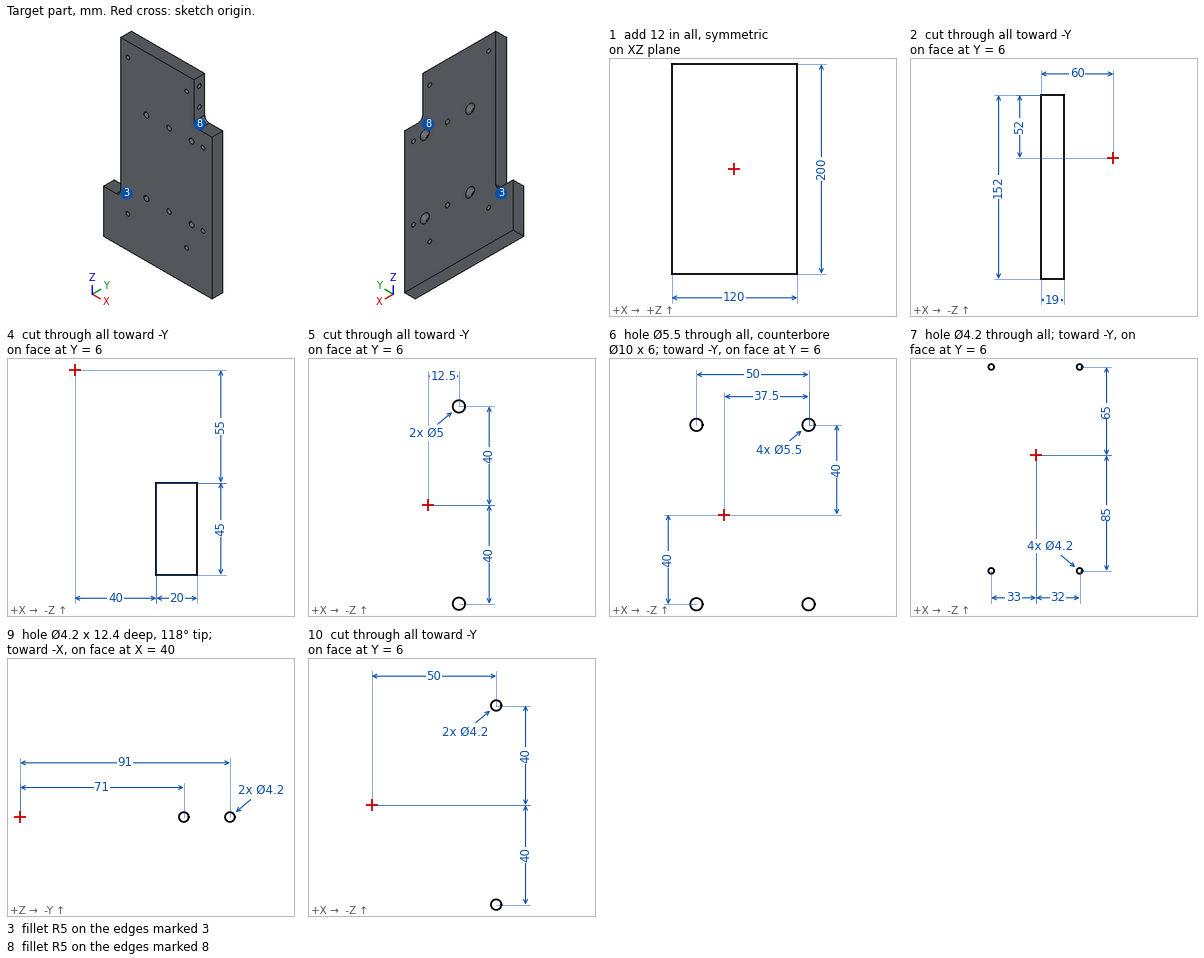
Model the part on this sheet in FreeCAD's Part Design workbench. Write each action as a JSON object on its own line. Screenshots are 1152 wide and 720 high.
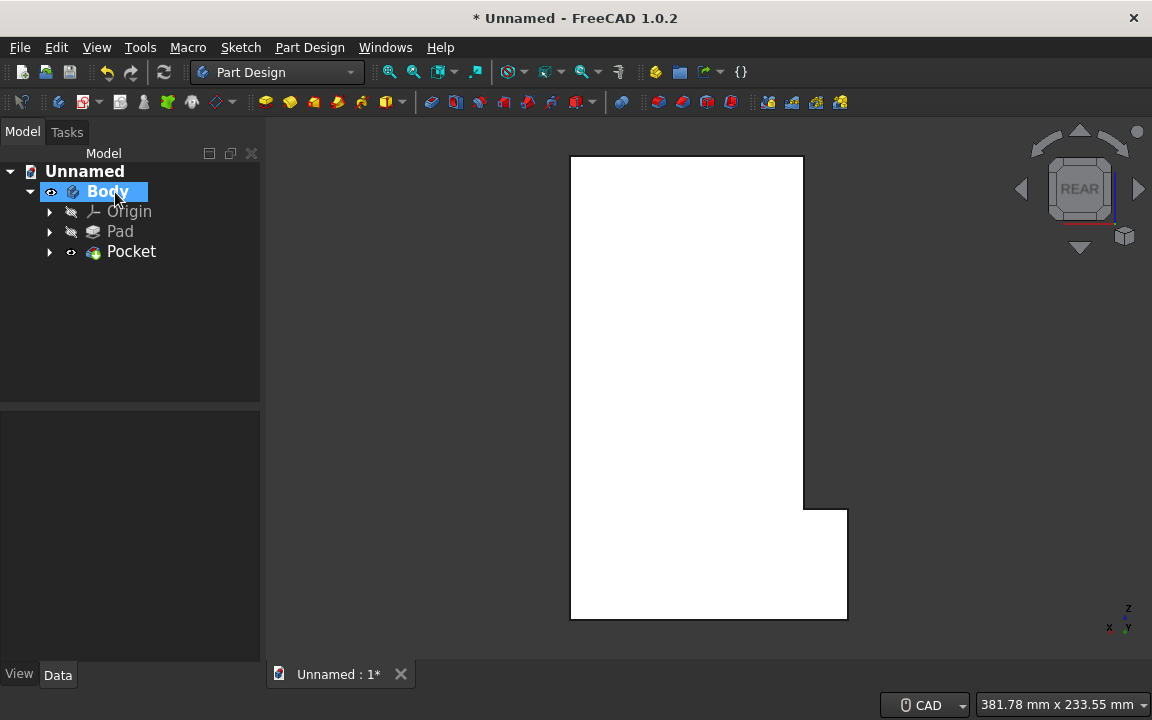
{"action": "key", "text": "0"}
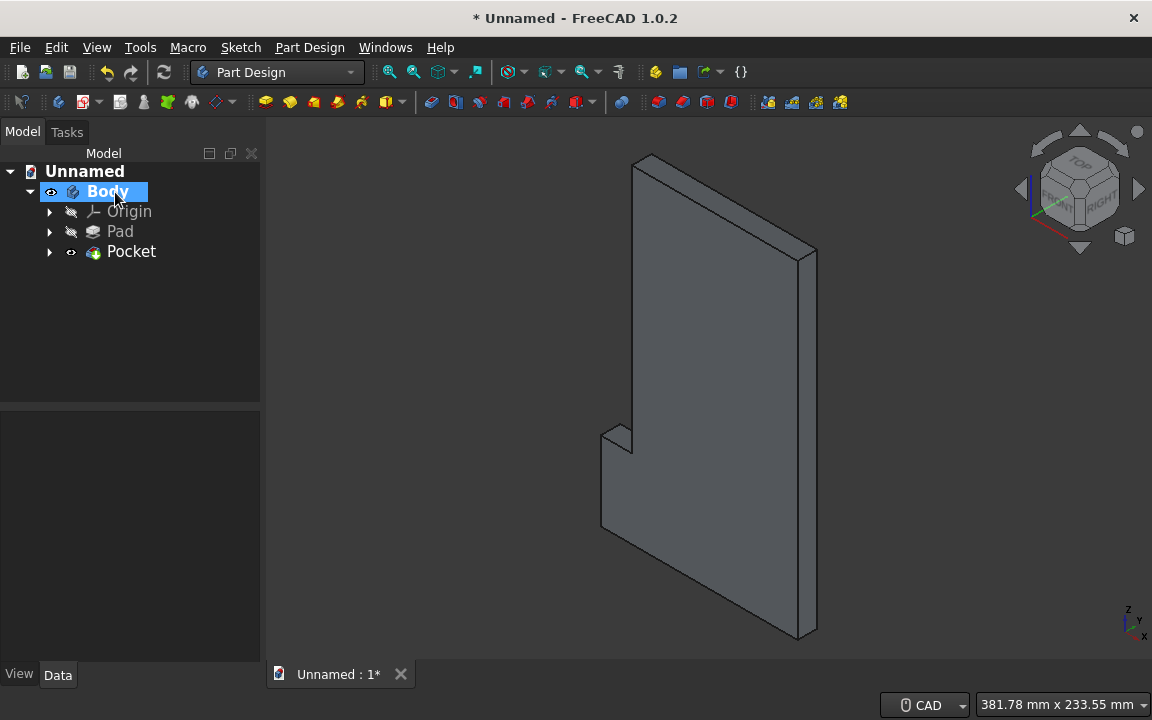
{"action": "key", "text": "2"}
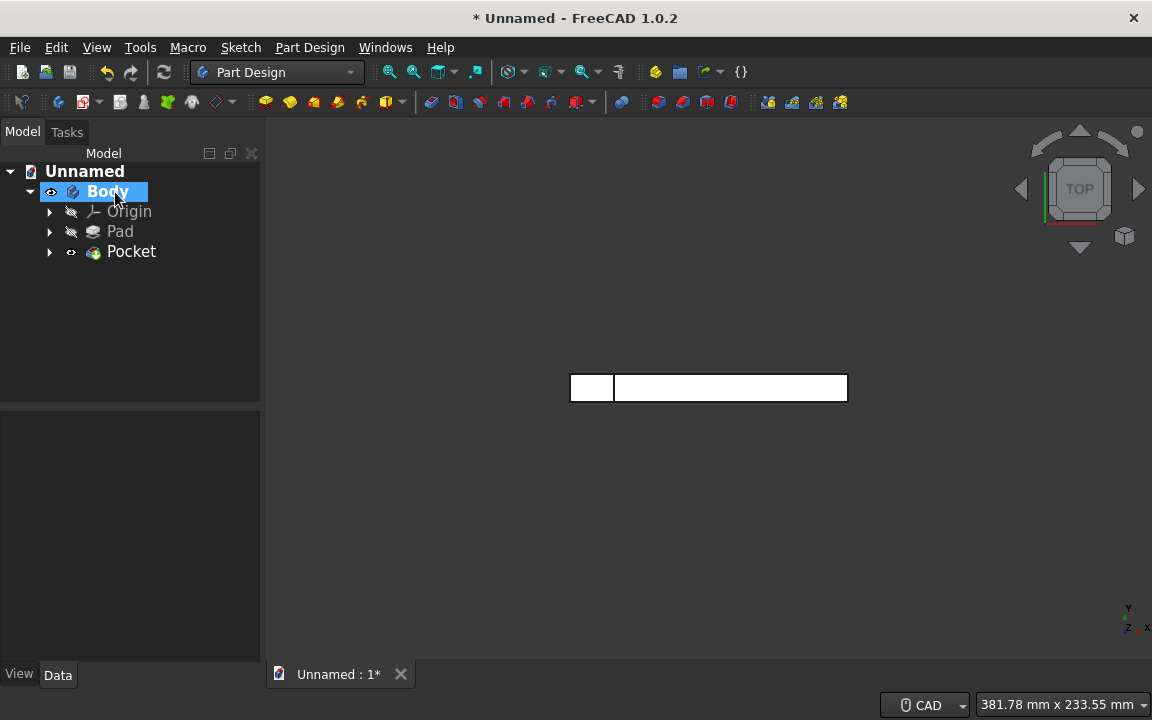
{"action": "left_click", "coordinate": [390, 72]}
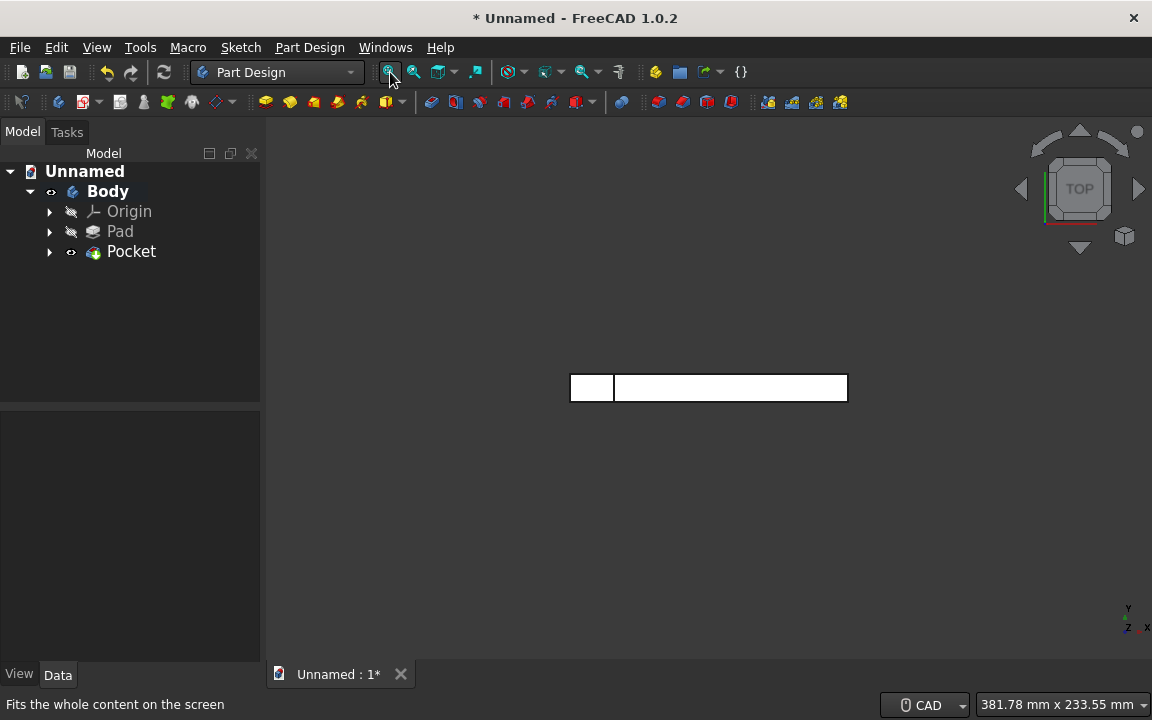
{"action": "key", "text": "1"}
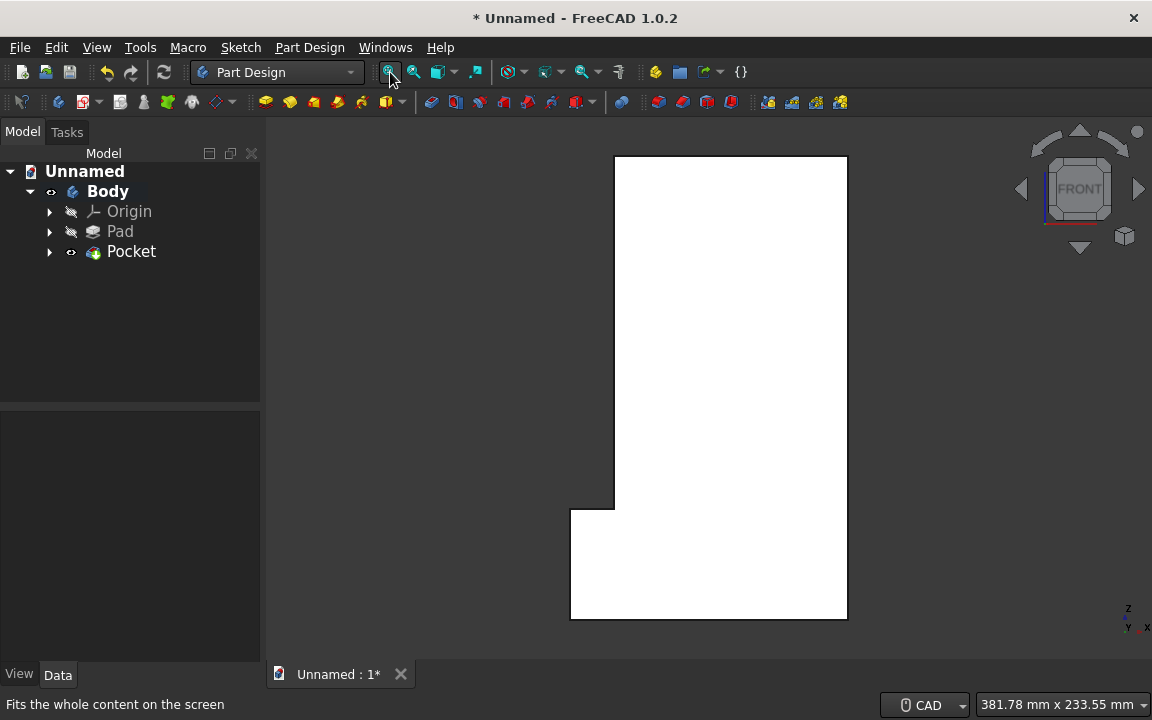
{"action": "key", "text": "3"}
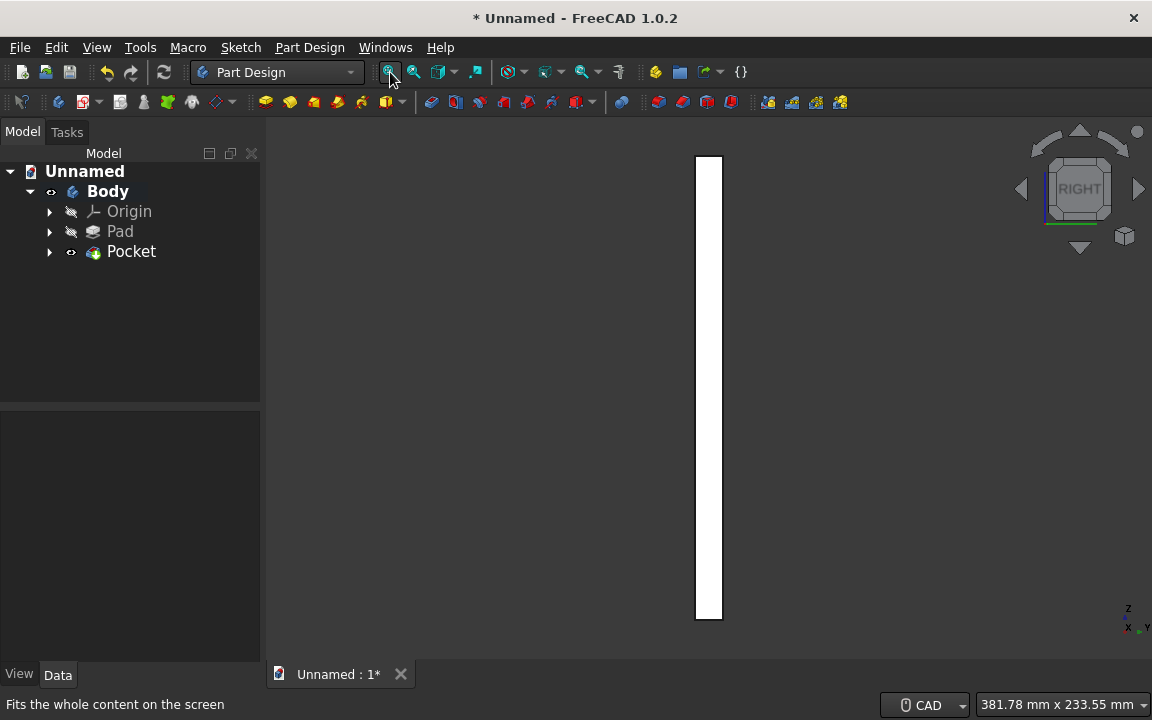
{"action": "key", "text": "5"}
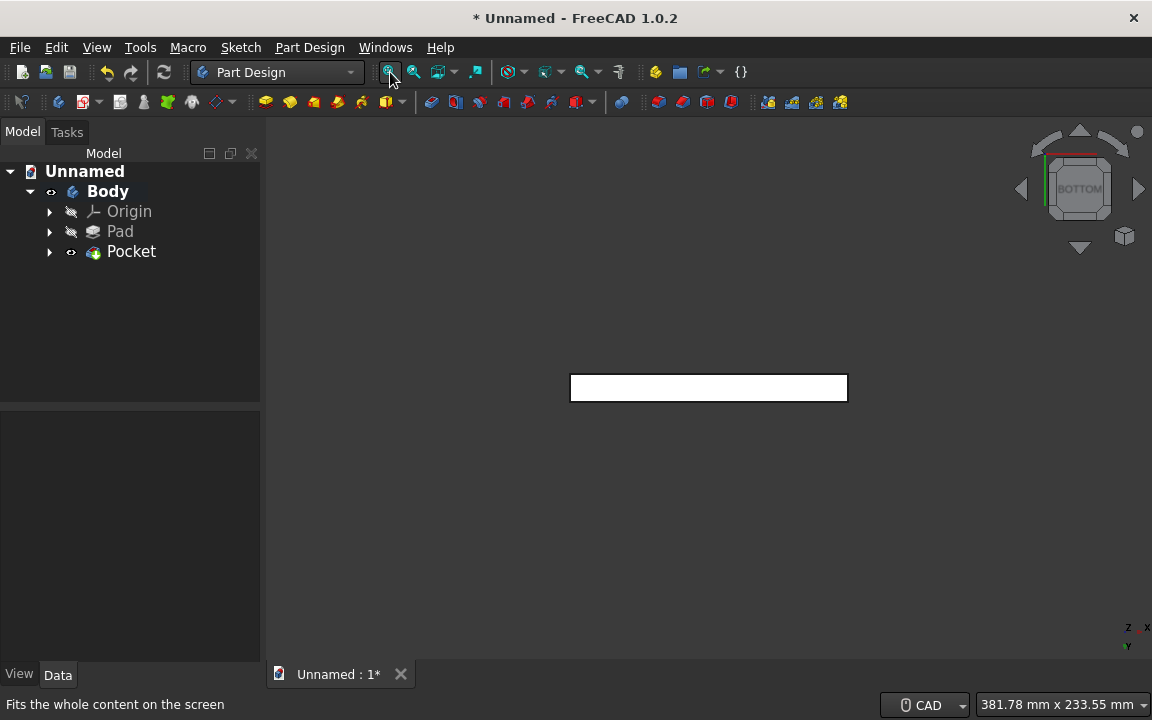
{"action": "left_click", "coordinate": [390, 72]}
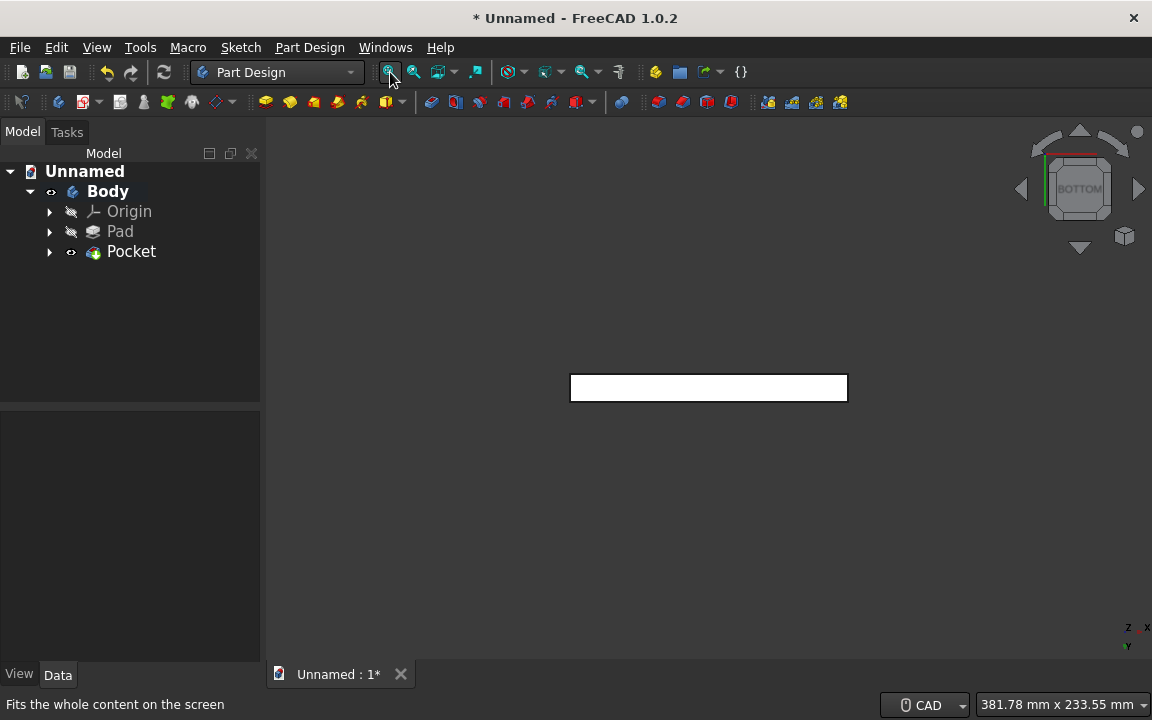
{"action": "key", "text": "4"}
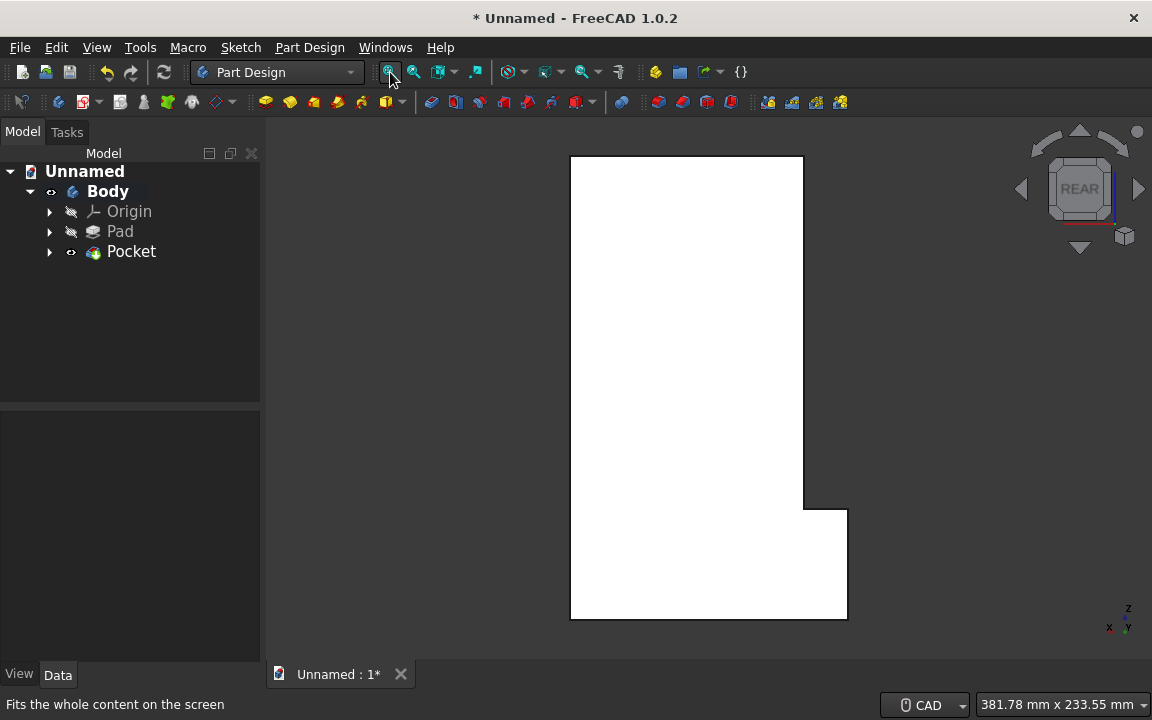
{"action": "key", "text": "6"}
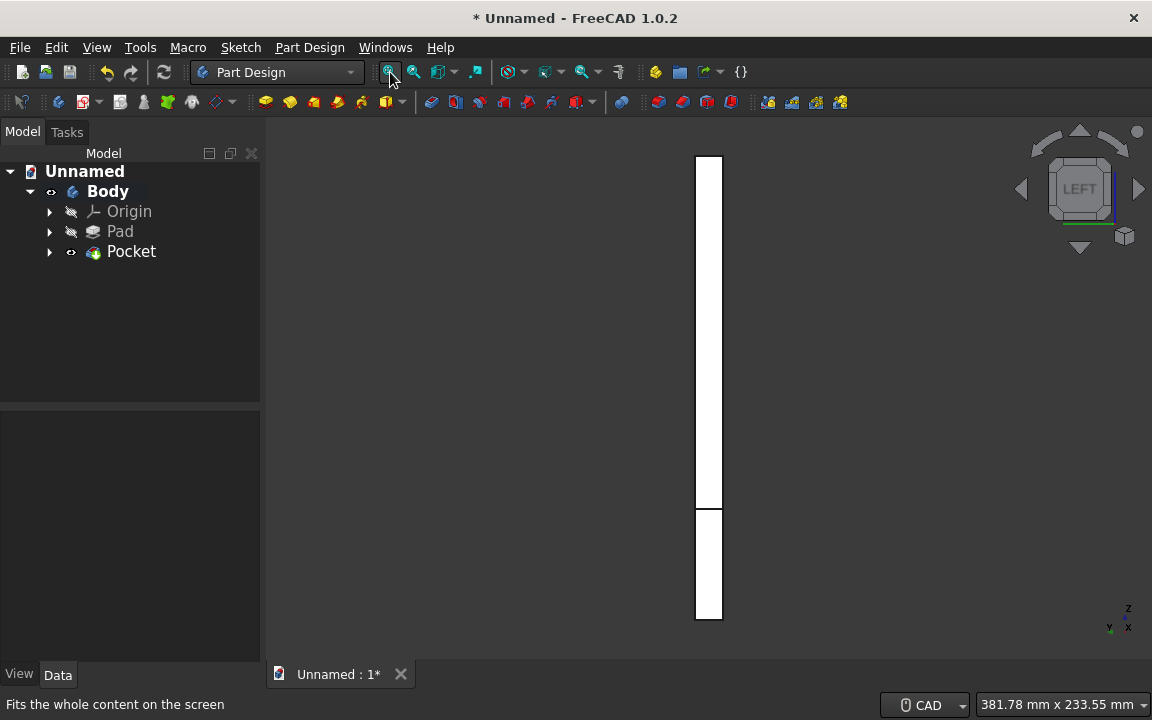
{"action": "key", "text": "v 3"}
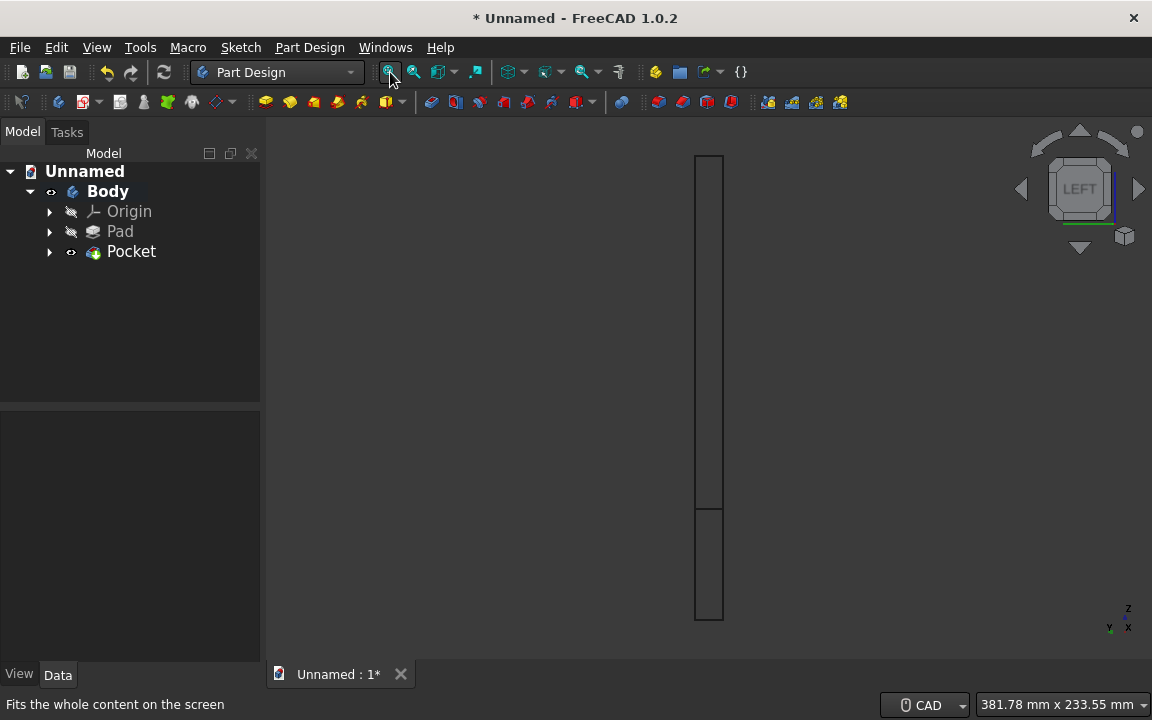
{"action": "key", "text": "0"}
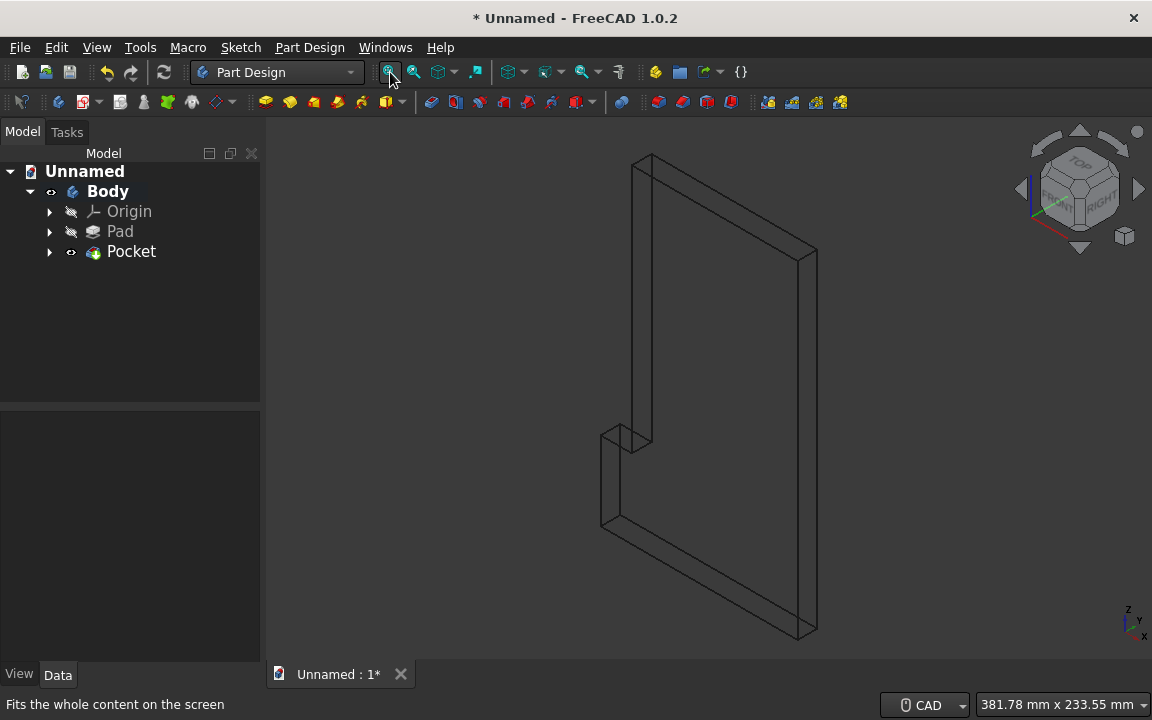
{"action": "left_click", "coordinate": [642, 447]}